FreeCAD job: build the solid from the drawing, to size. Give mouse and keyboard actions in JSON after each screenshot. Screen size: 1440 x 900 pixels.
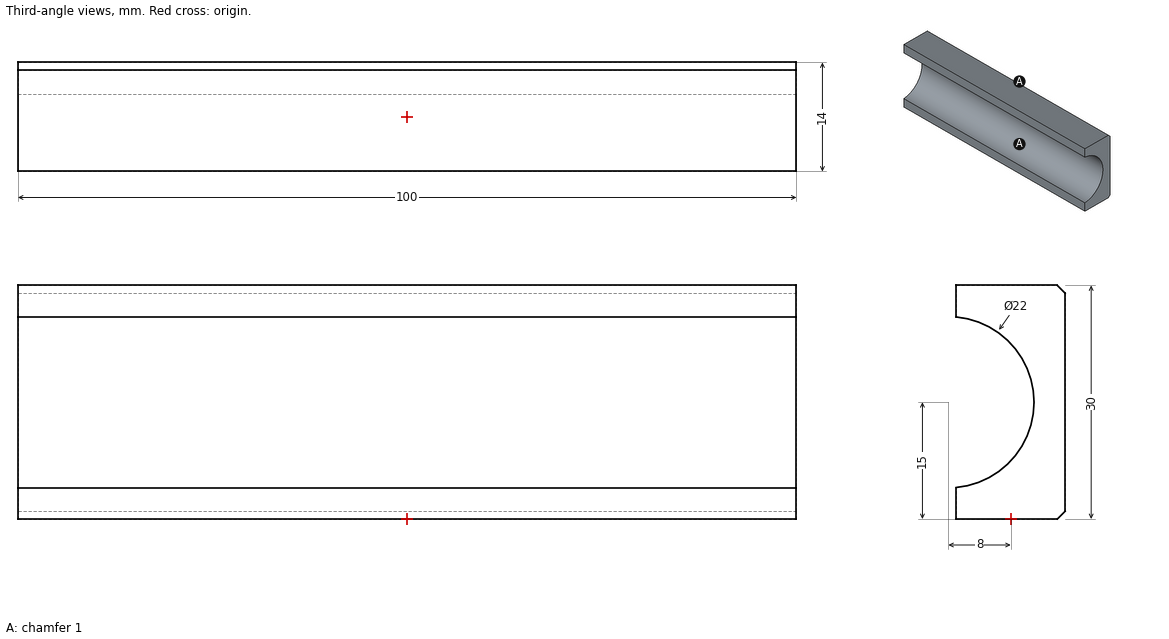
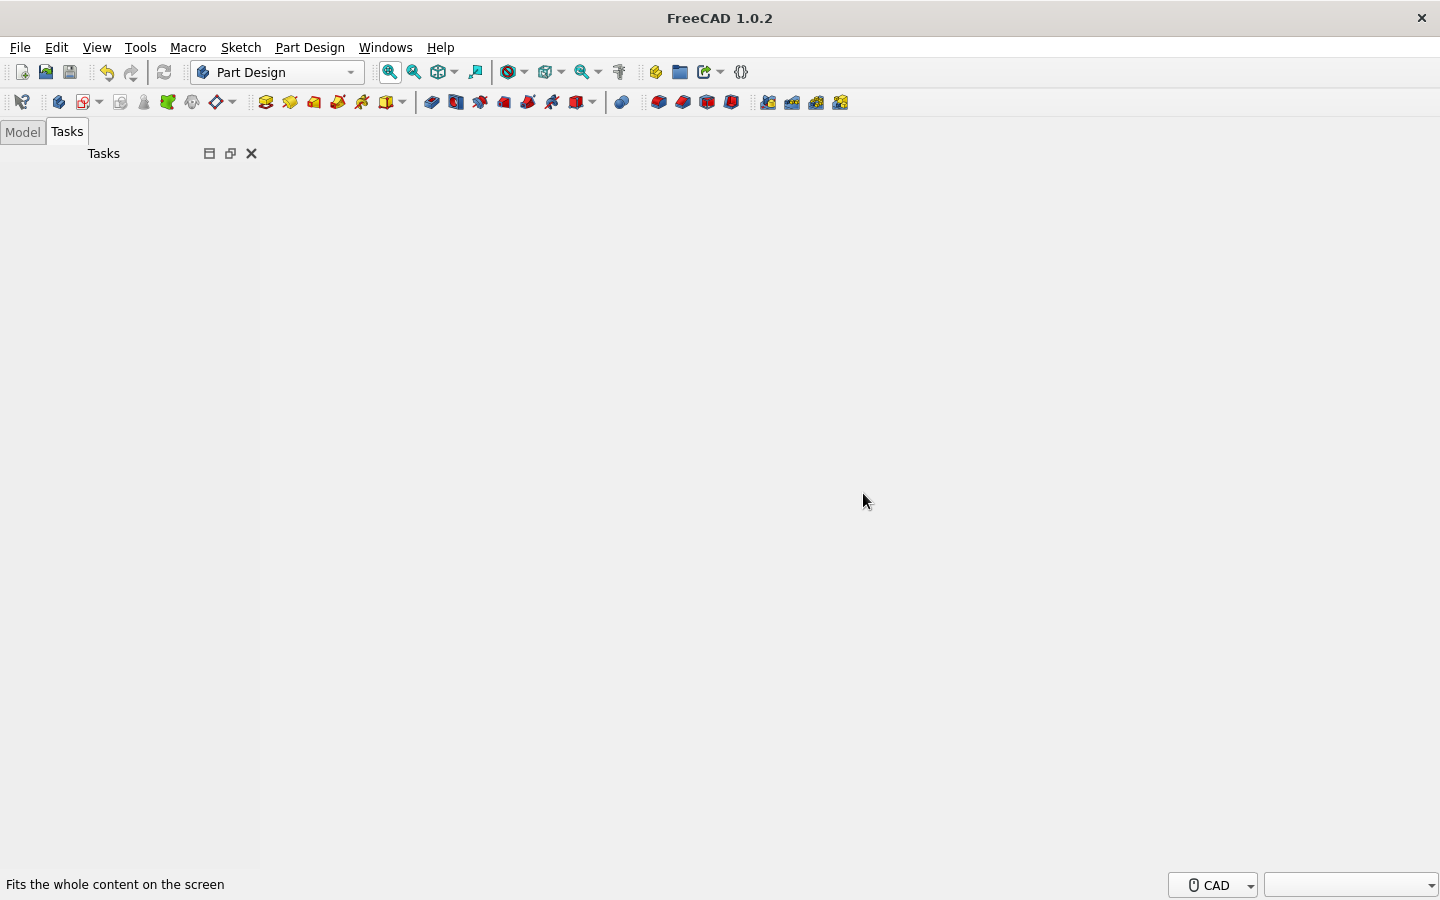
{"action": "key", "text": "ctrl+n"}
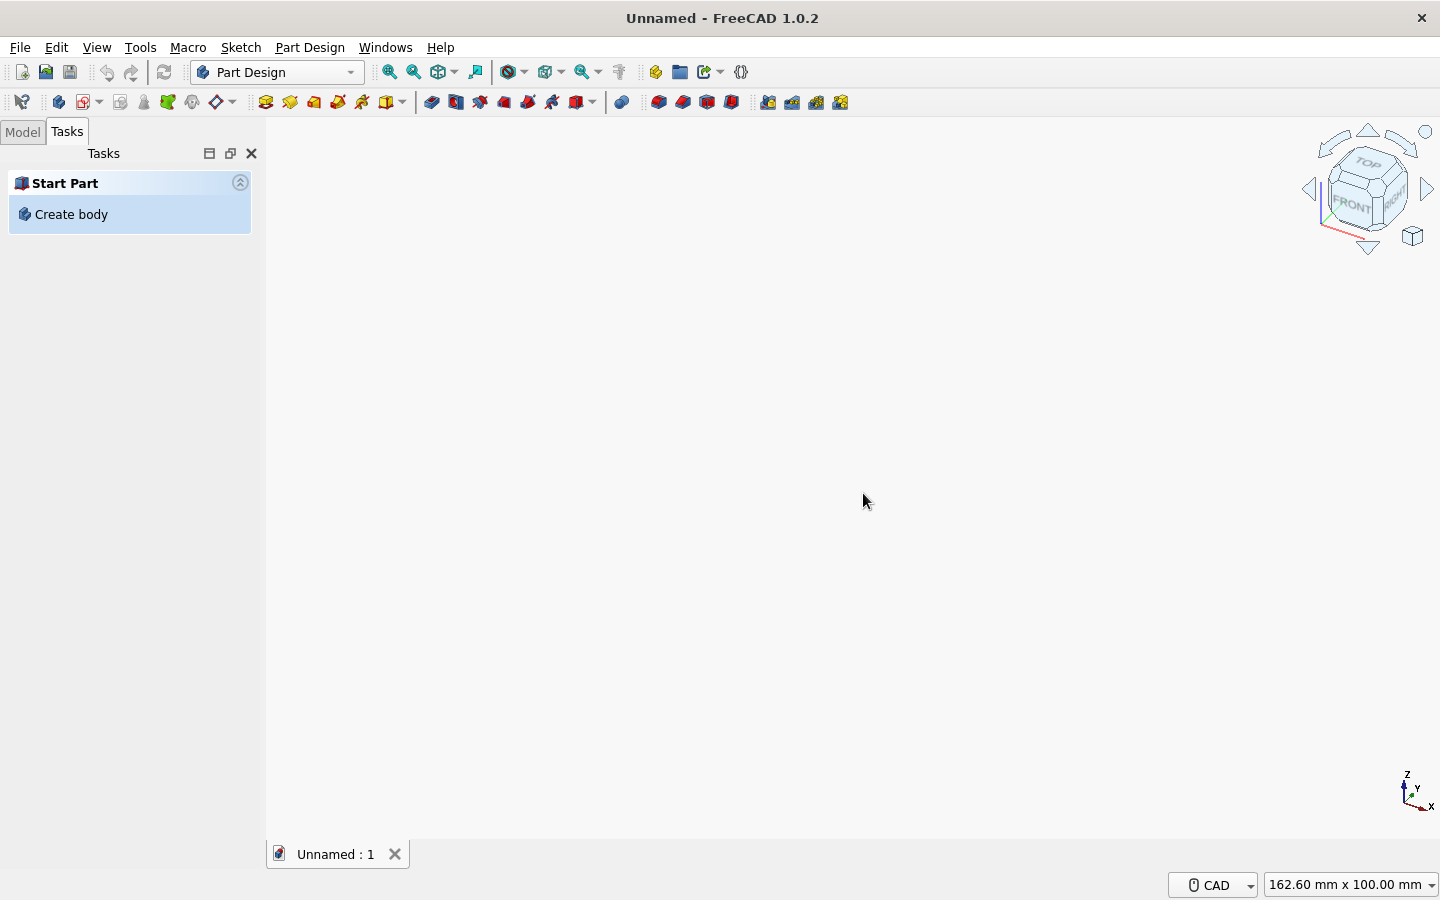
{"action": "left_click", "coordinate": [84, 102]}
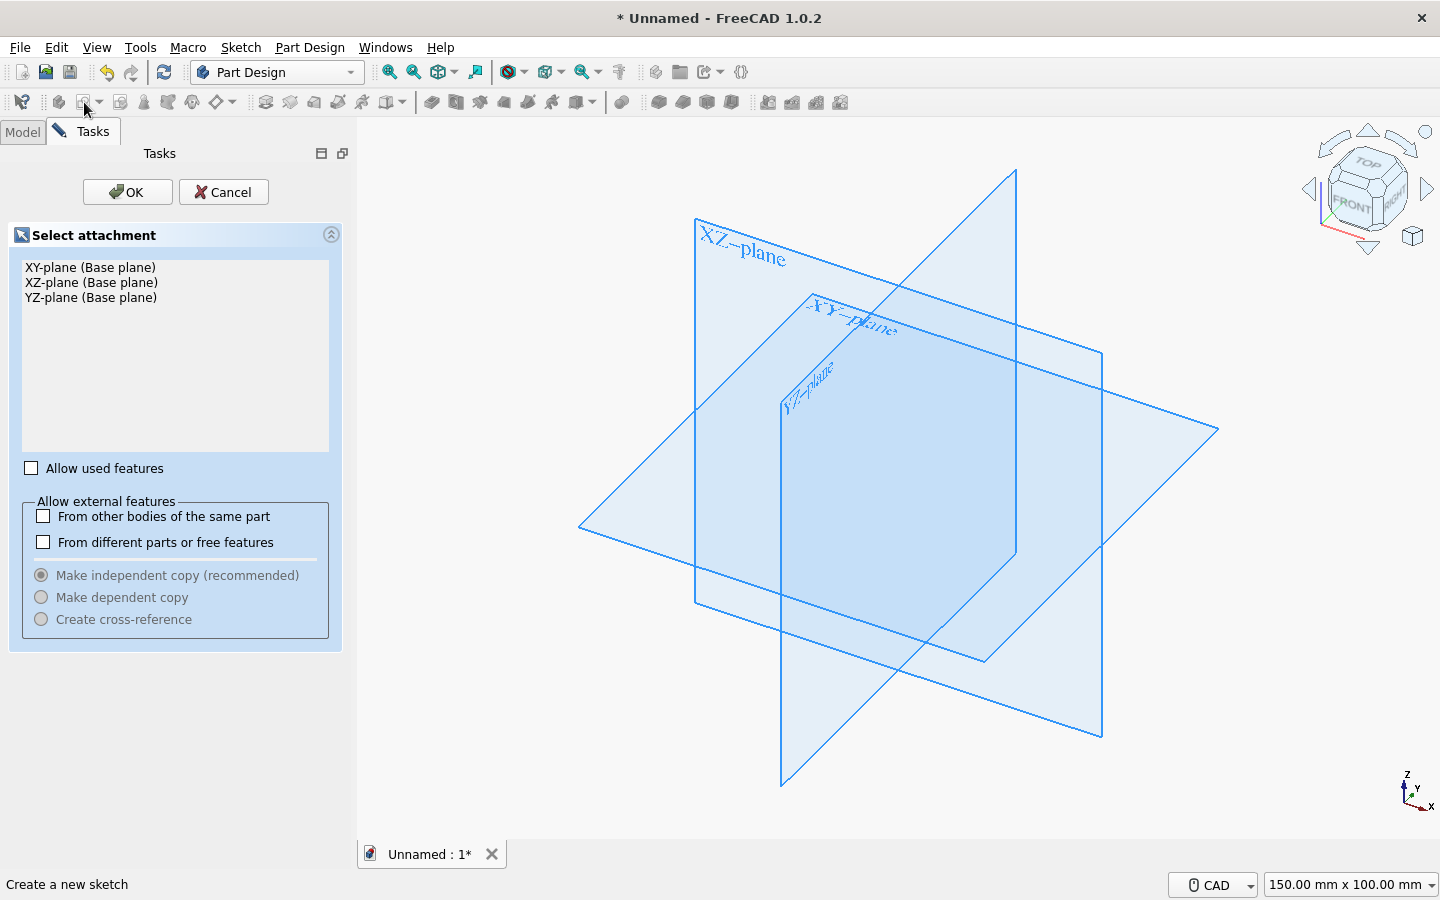
{"action": "left_click", "coordinate": [82, 268]}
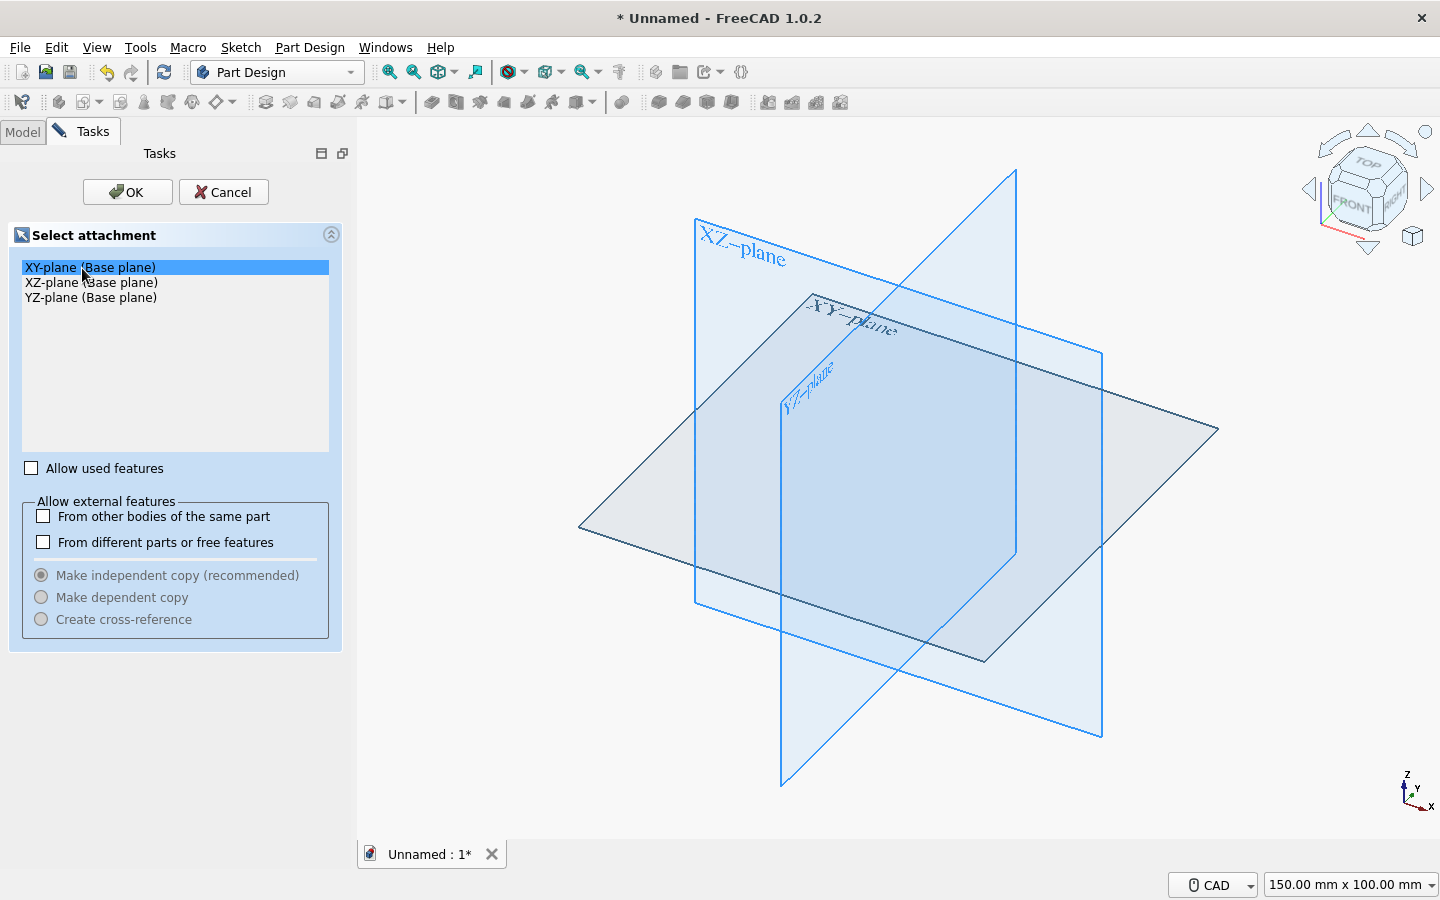
{"action": "left_click", "coordinate": [128, 192]}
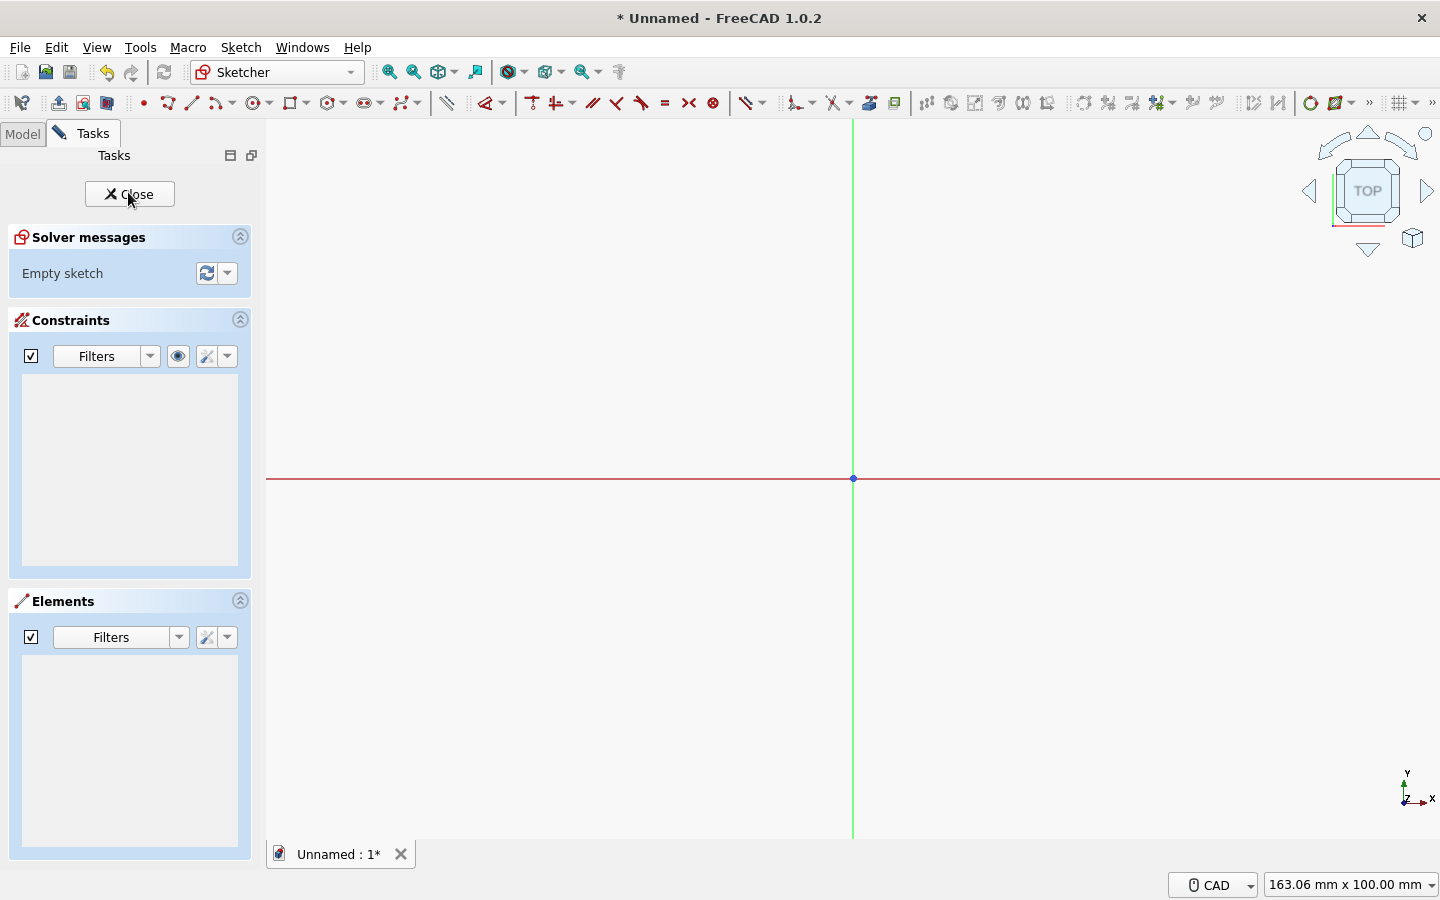
{"action": "key", "text": "g v"}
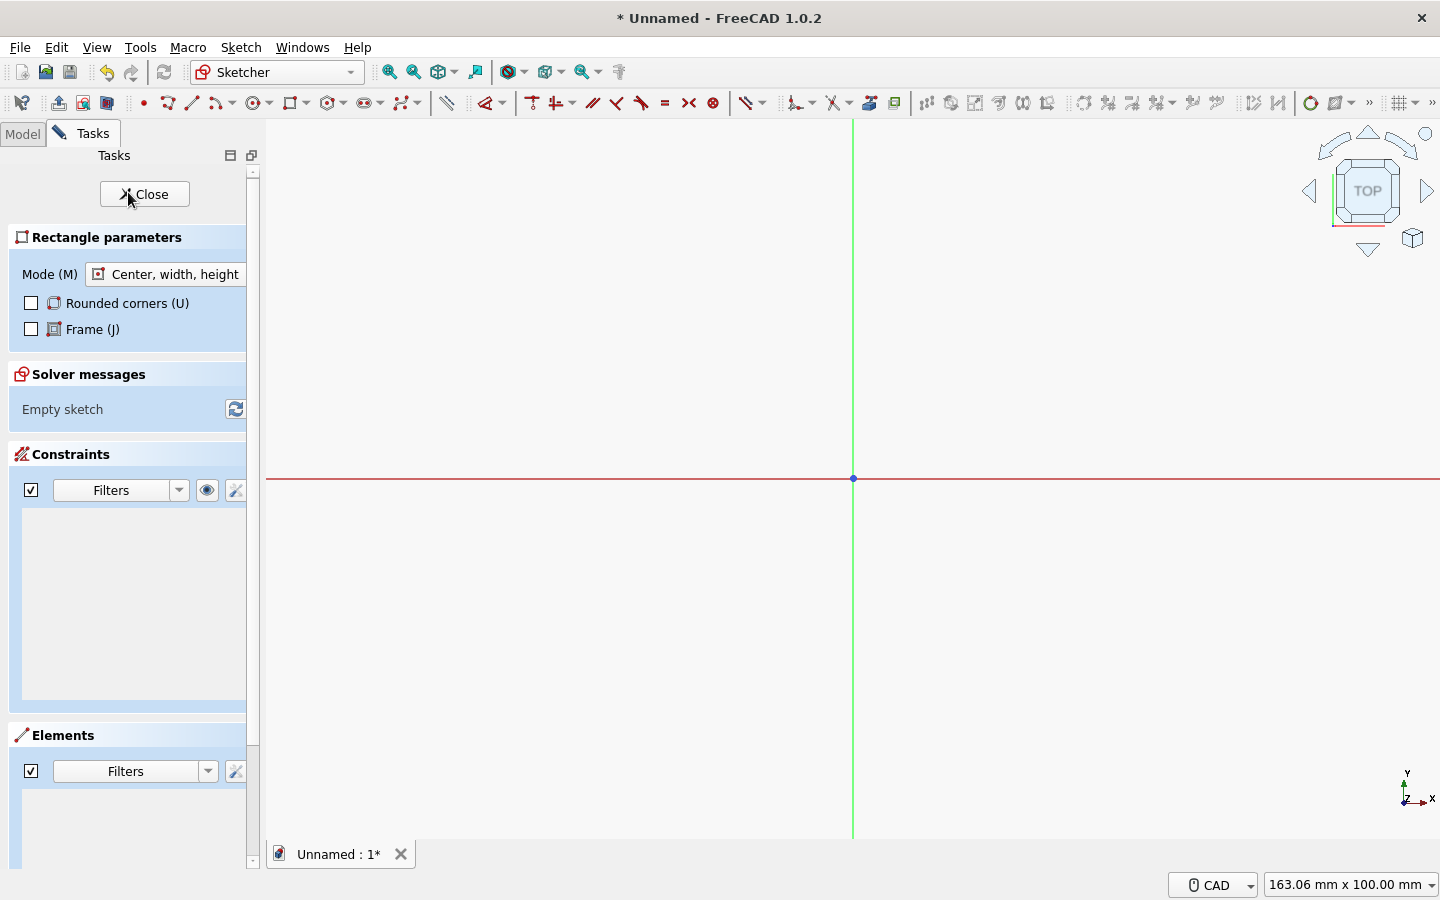
{"action": "left_click", "coordinate": [853, 479]}
{"action": "left_click", "coordinate": [1213, 429]}
{"action": "key", "text": "Escape"}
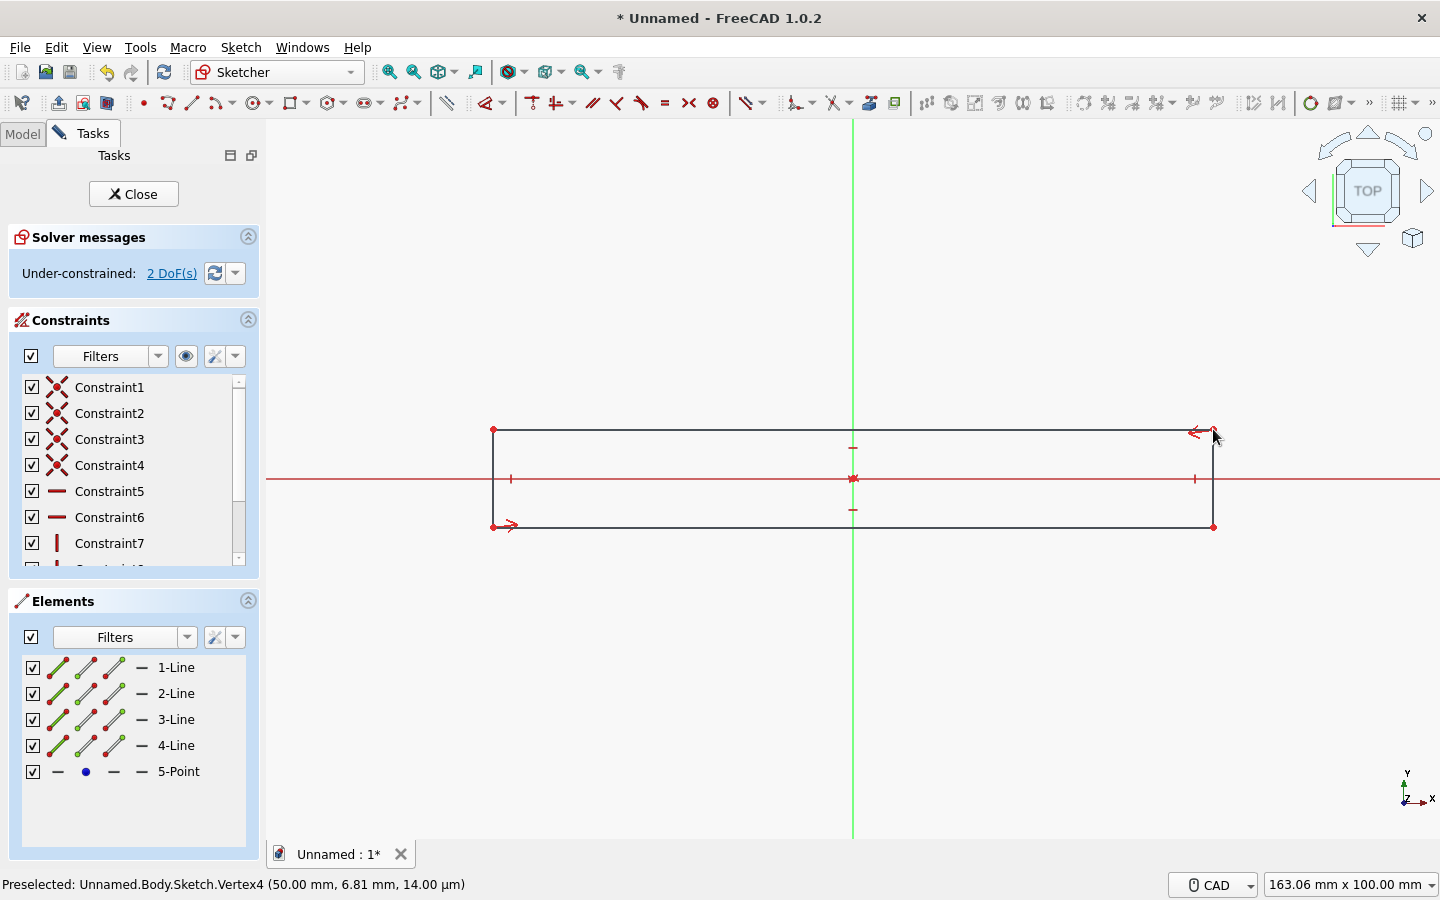
{"action": "left_click", "coordinate": [1213, 499]}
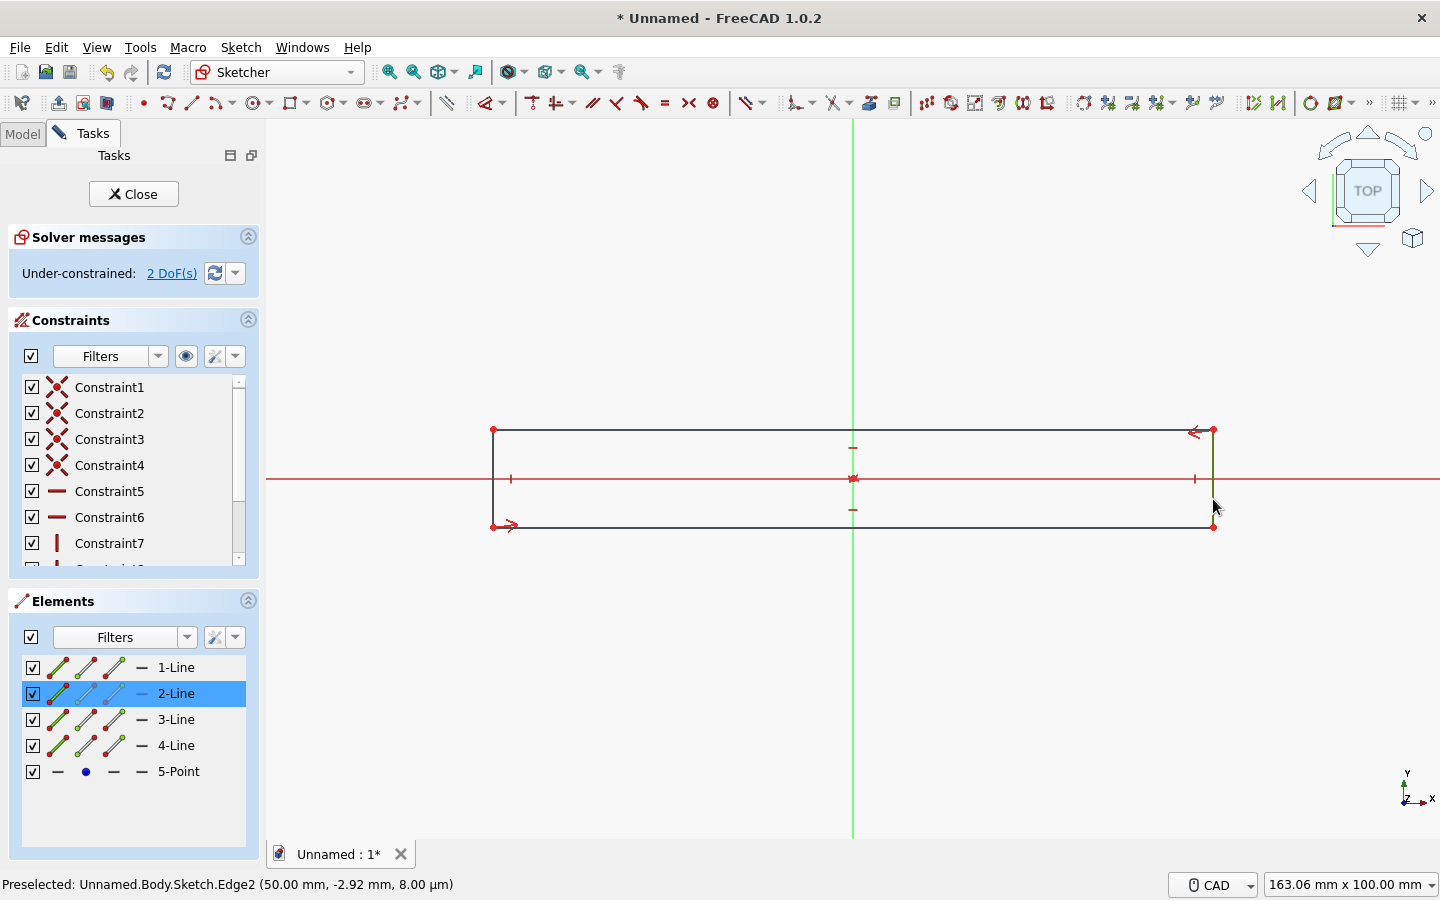
{"action": "key", "text": "i"}